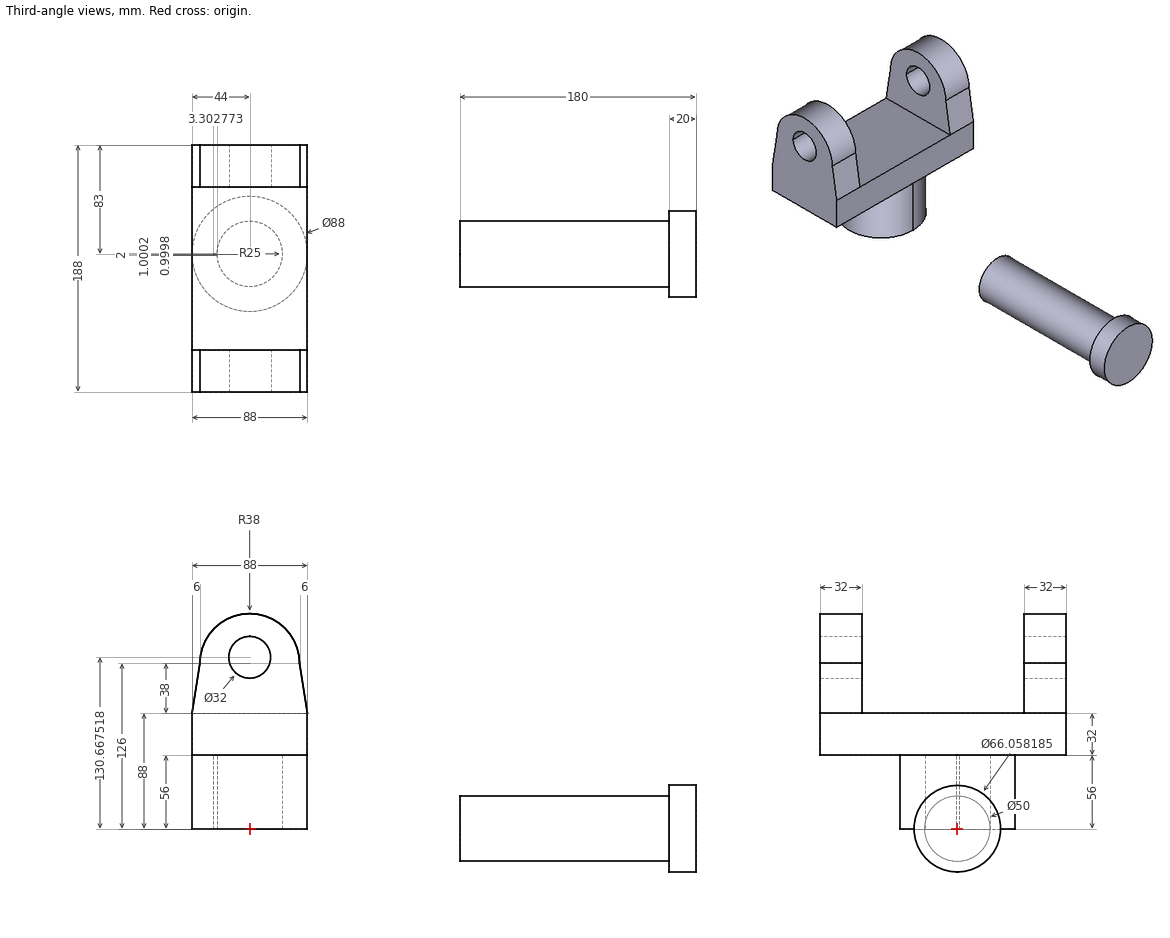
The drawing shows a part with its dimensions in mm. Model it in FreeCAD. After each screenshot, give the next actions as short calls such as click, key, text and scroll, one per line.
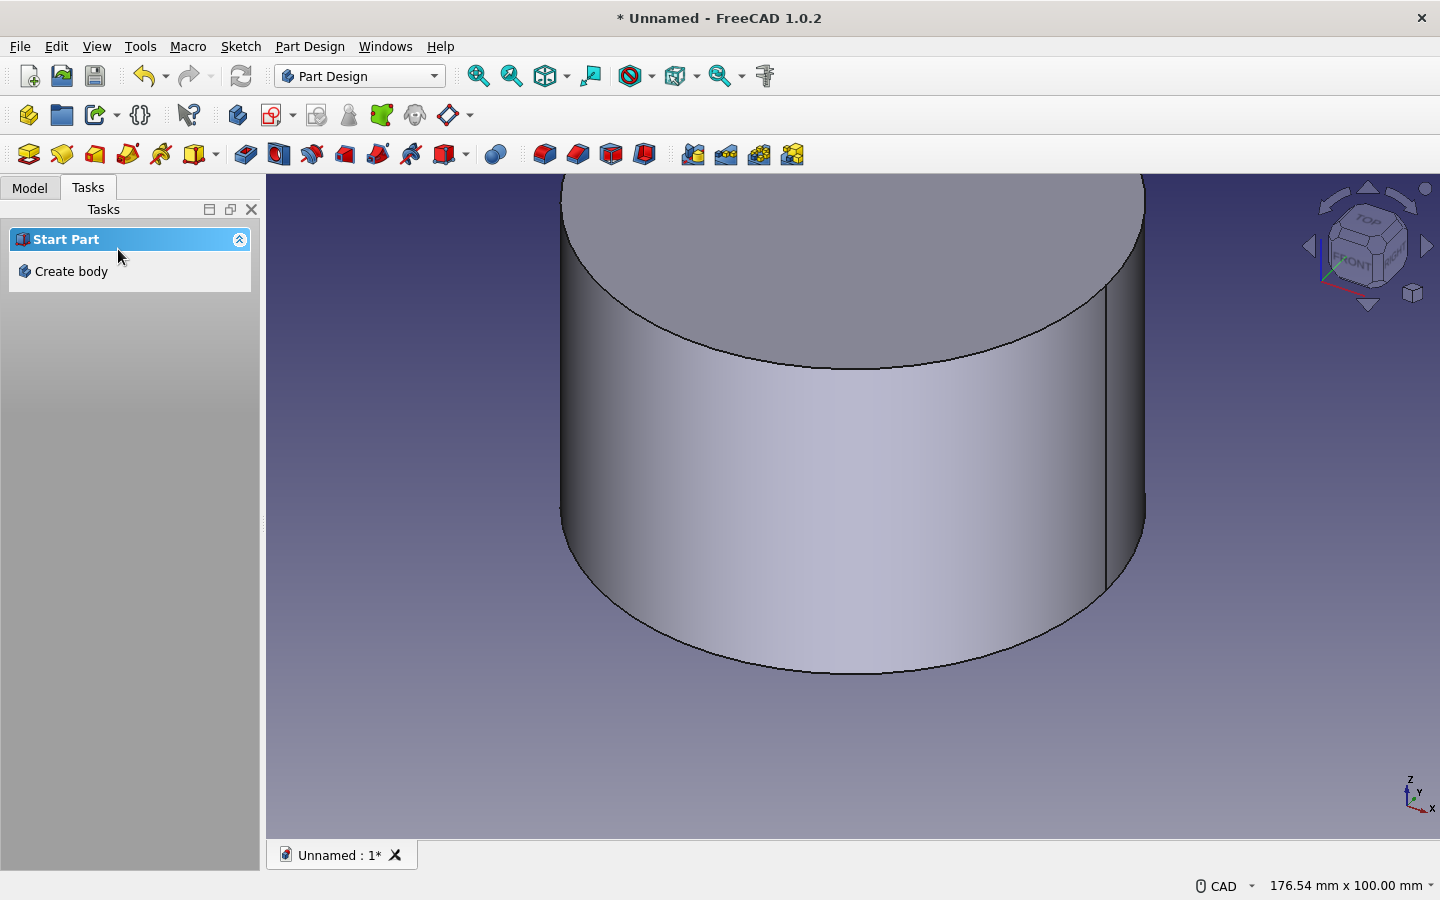
click(479, 76)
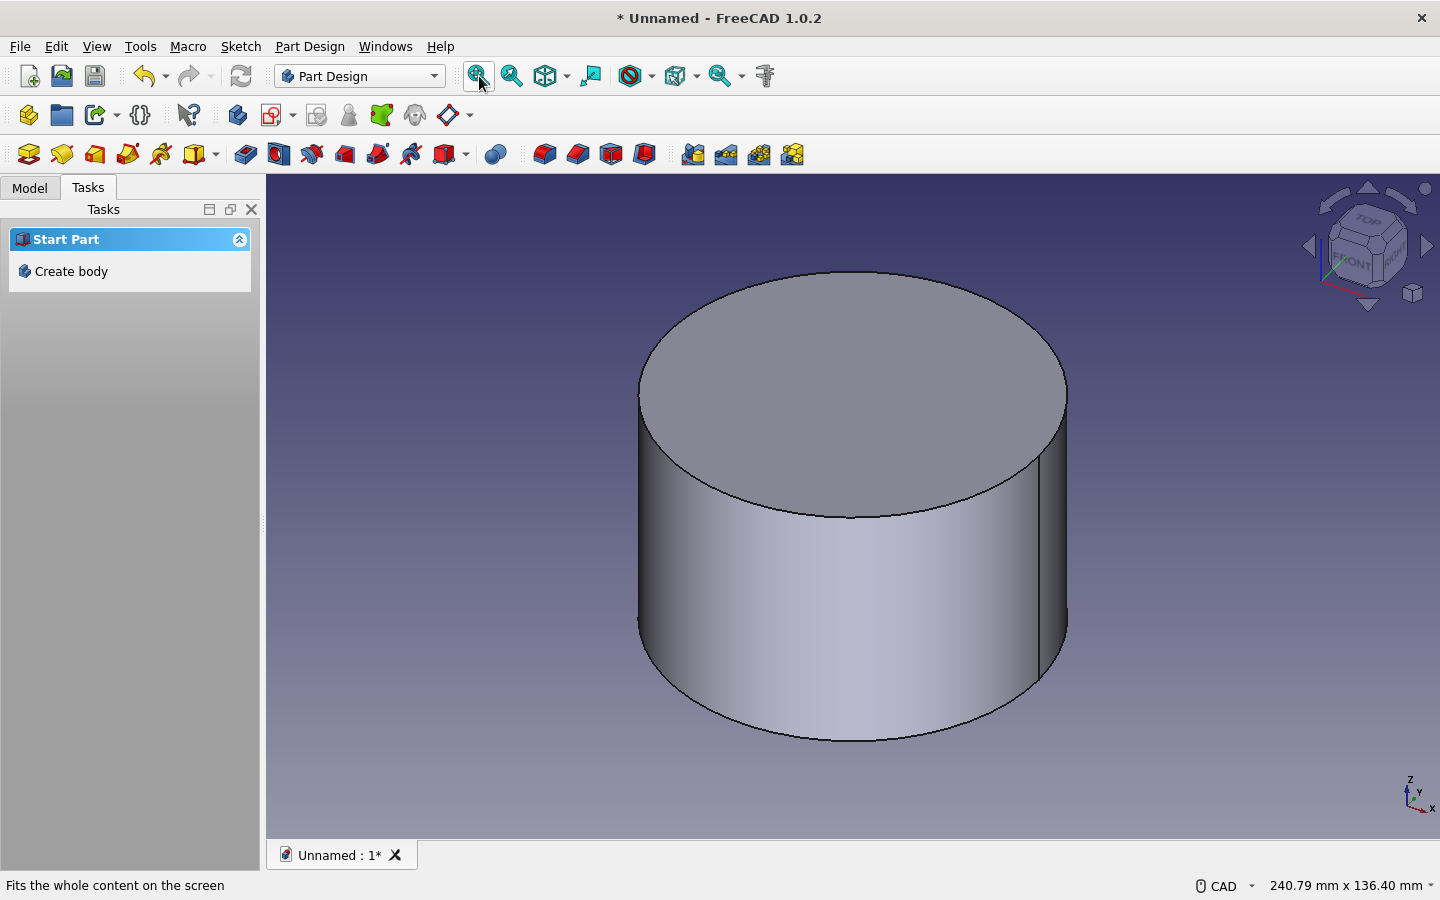
key(5)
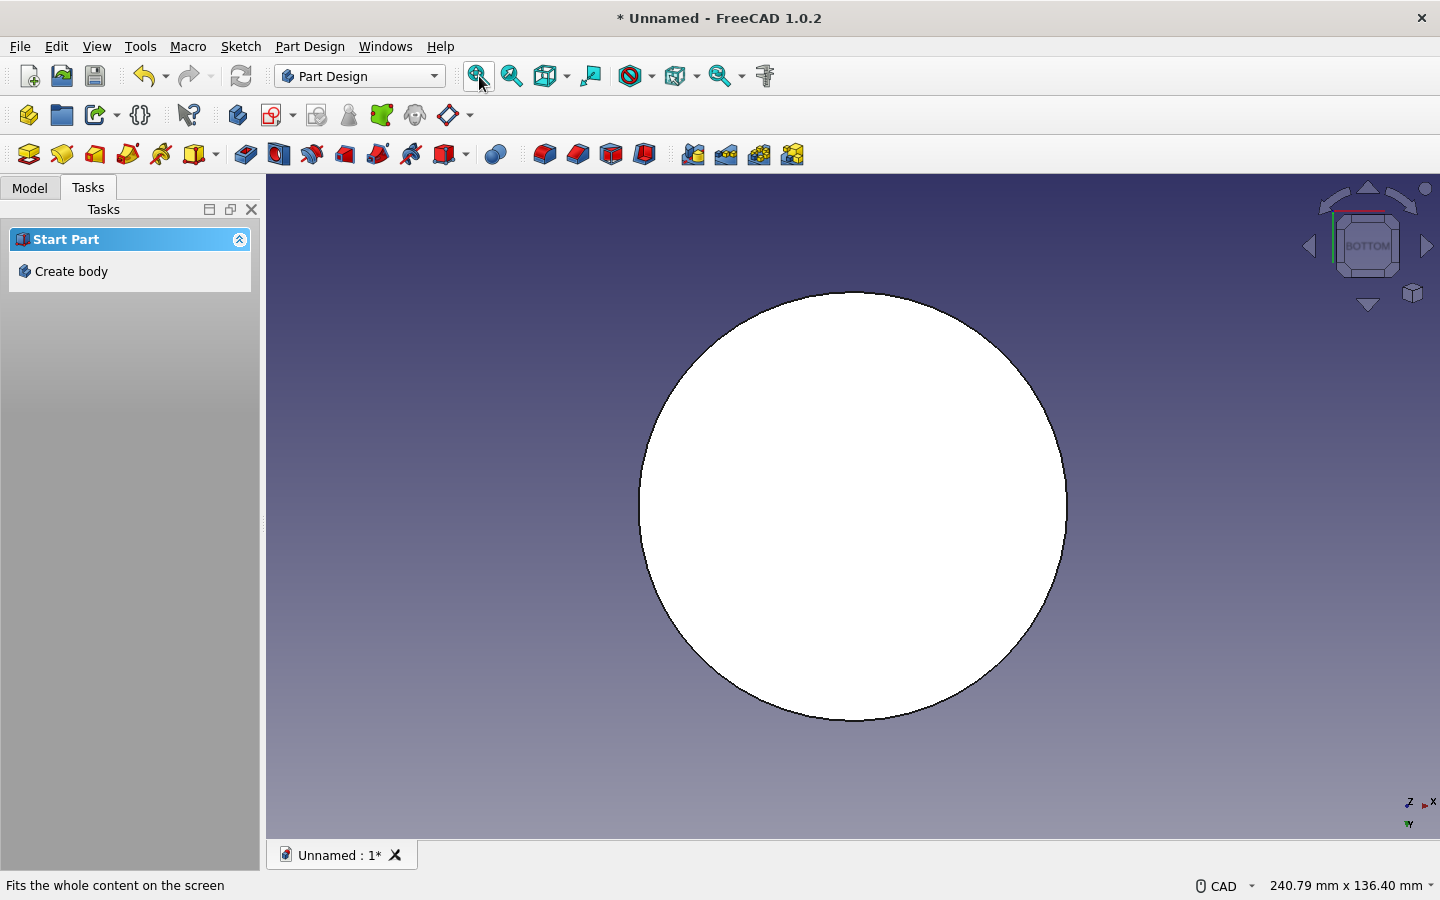
click(853, 505)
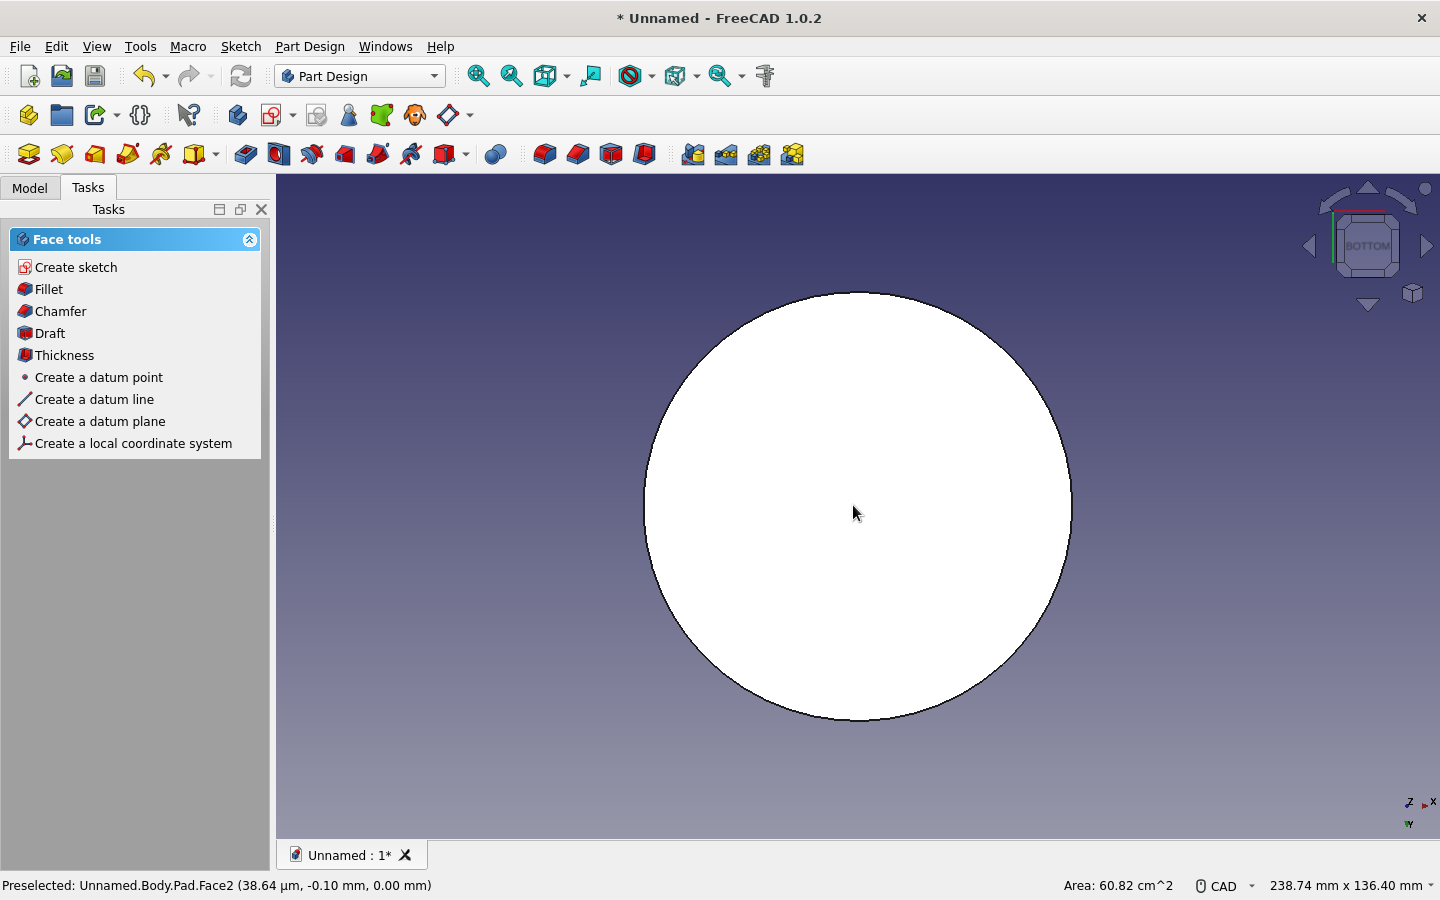
click(270, 116)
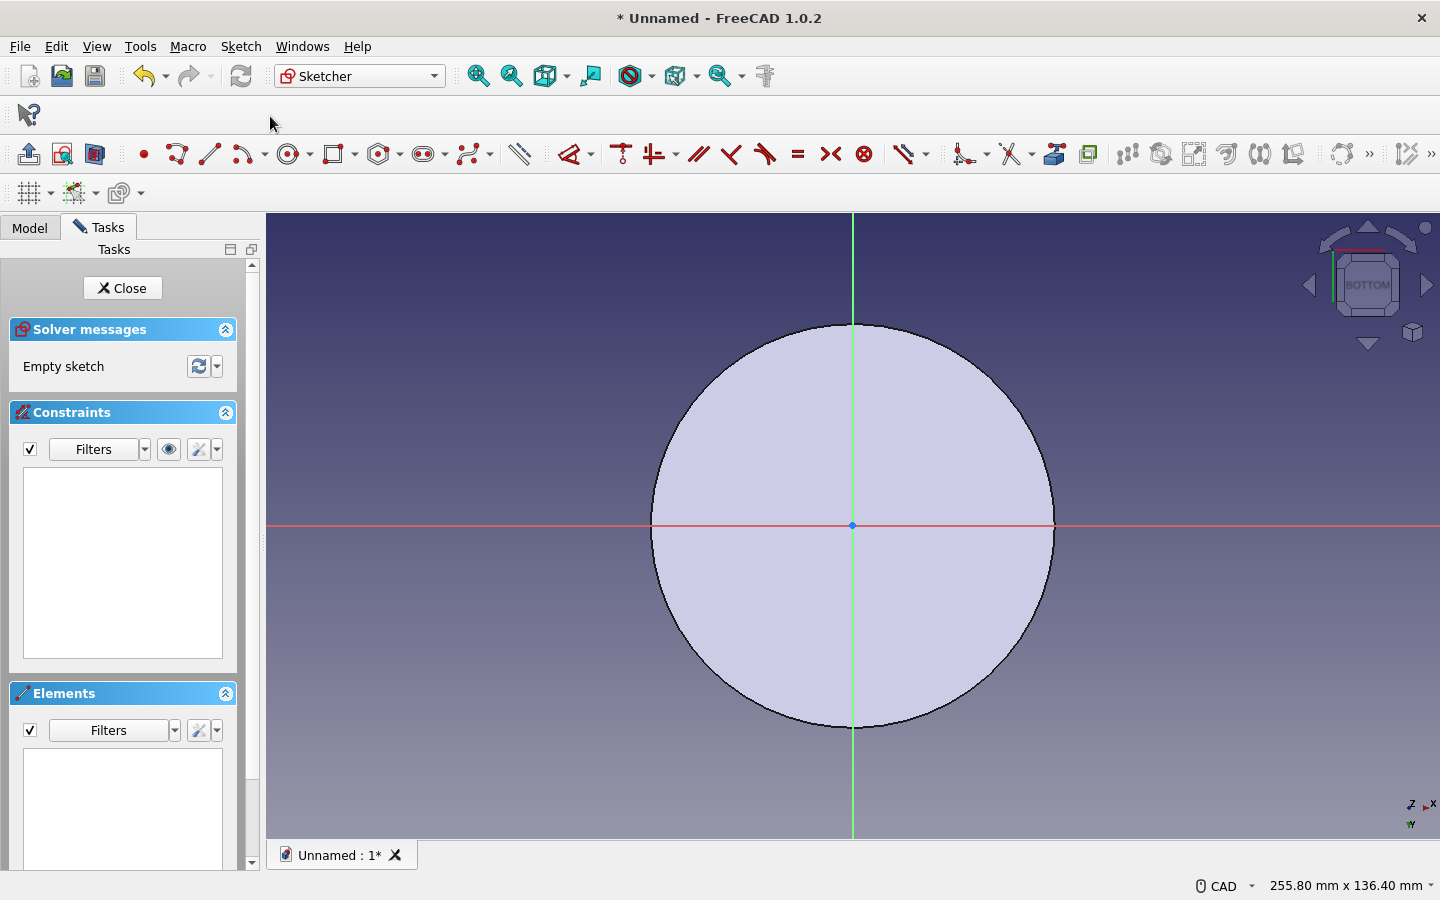
scroll(881, 526, up, 5)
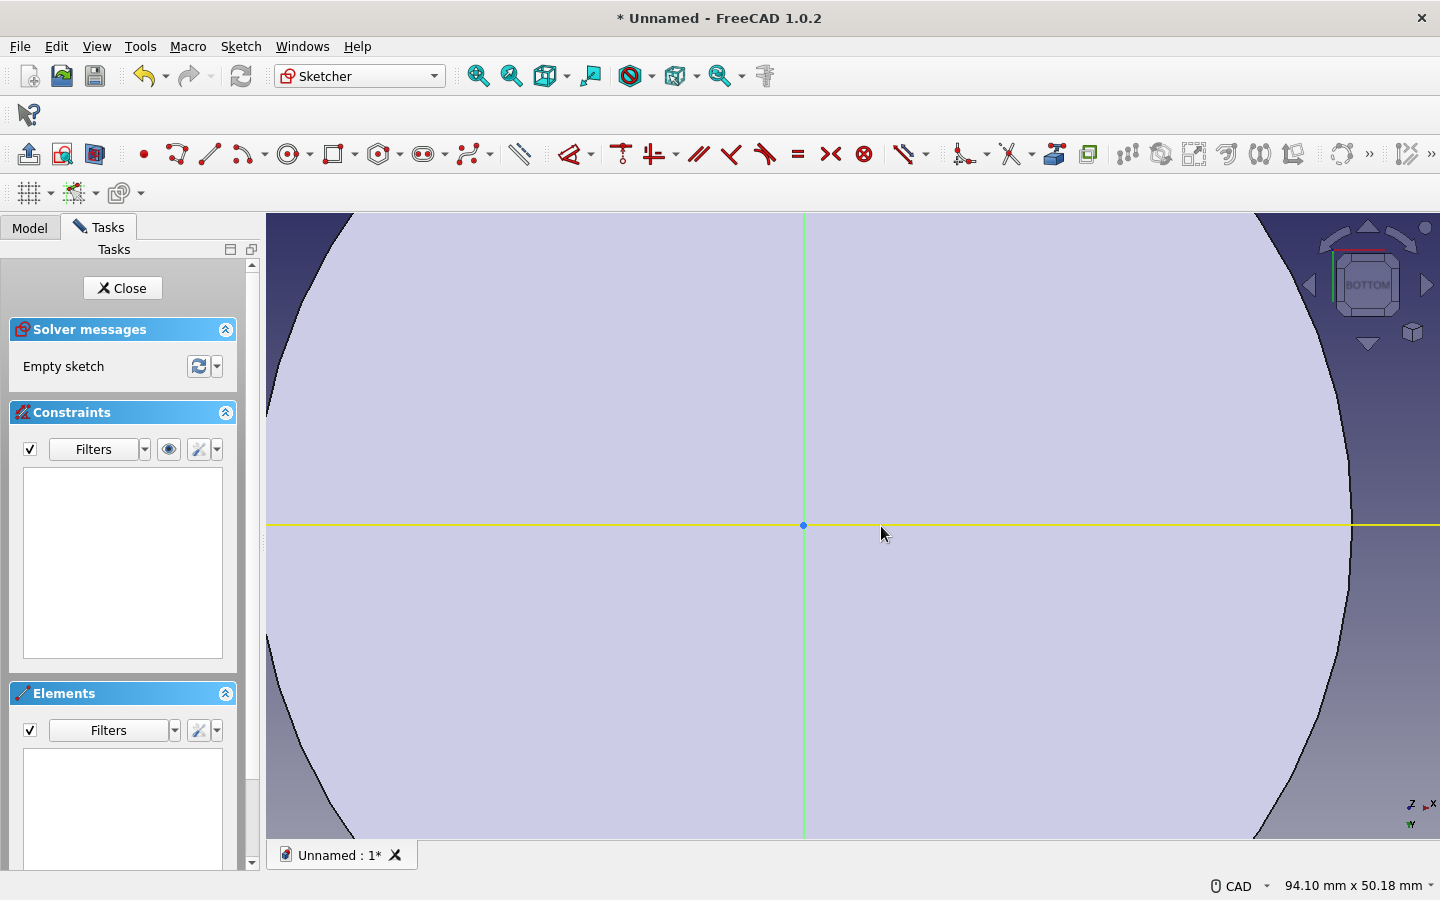
click(177, 154)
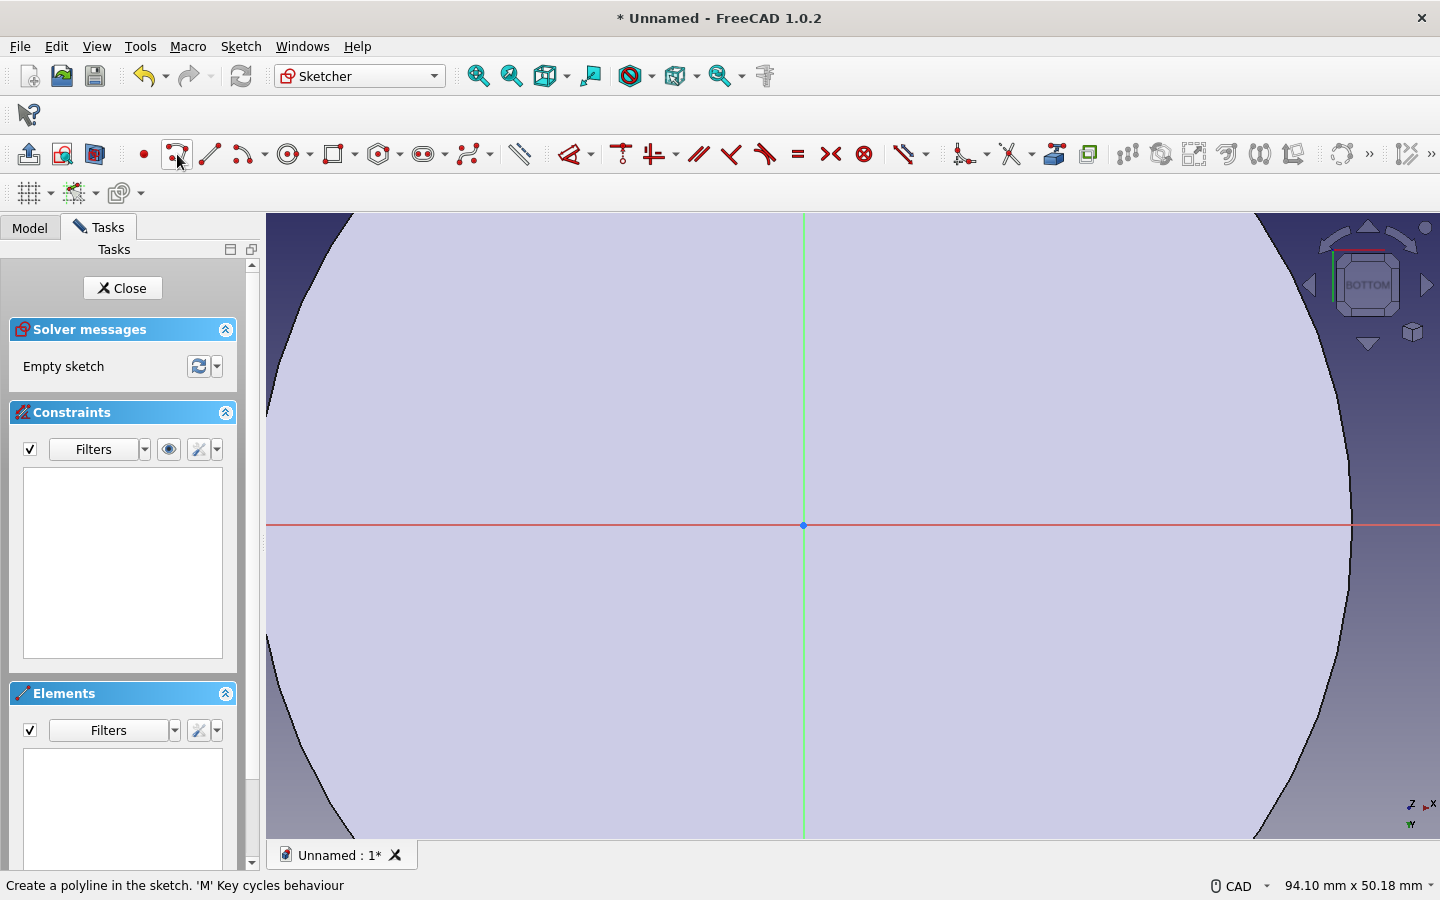
scroll(492, 513, up, 2)